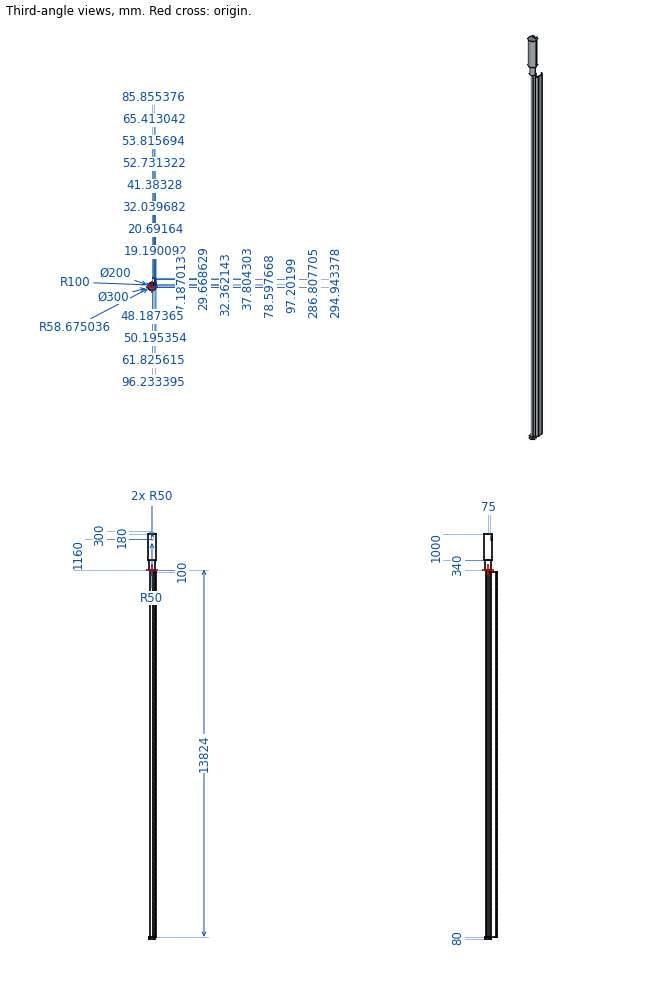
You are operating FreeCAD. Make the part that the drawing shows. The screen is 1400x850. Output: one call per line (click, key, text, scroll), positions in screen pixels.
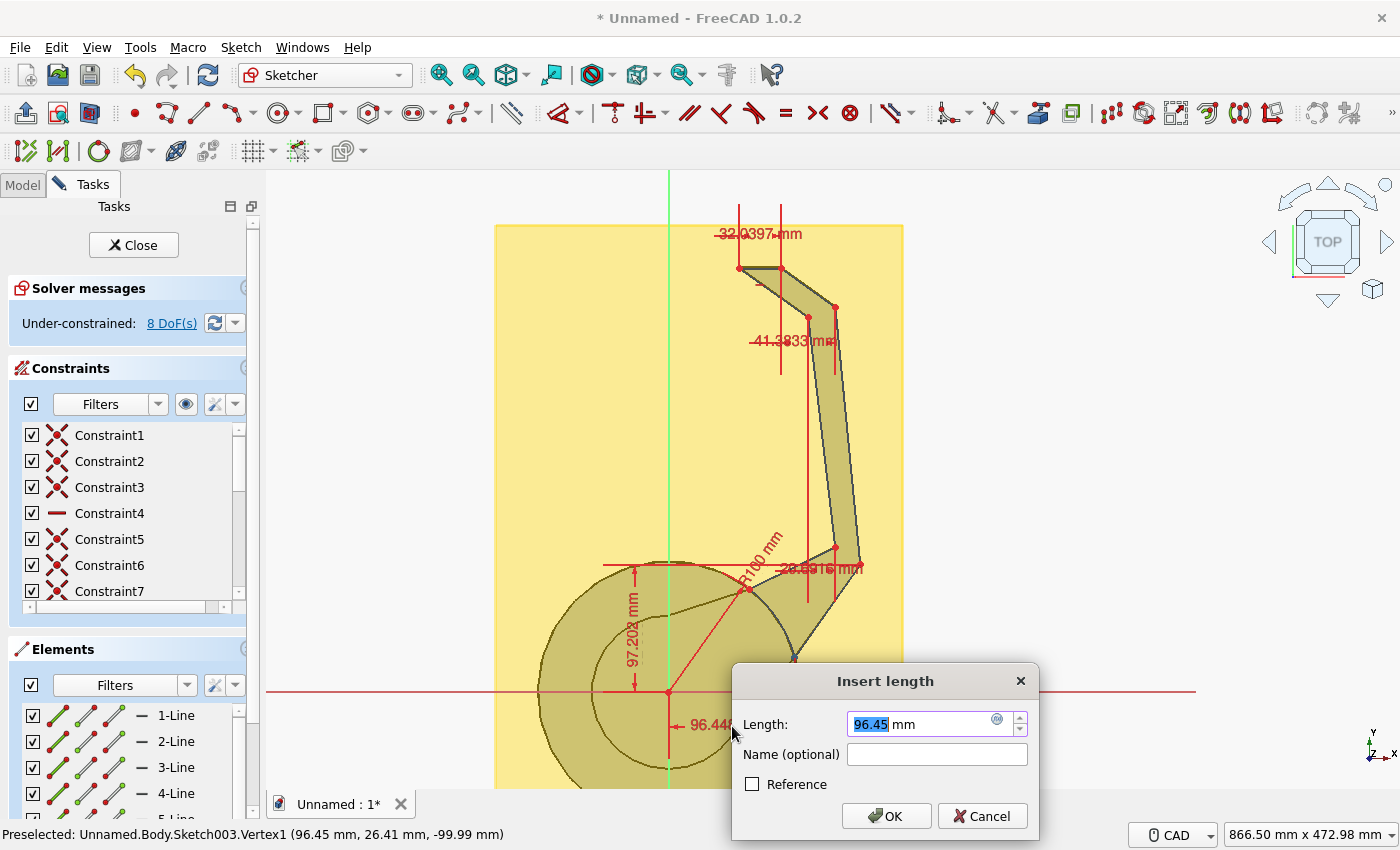
text(96.233395)
key(Return)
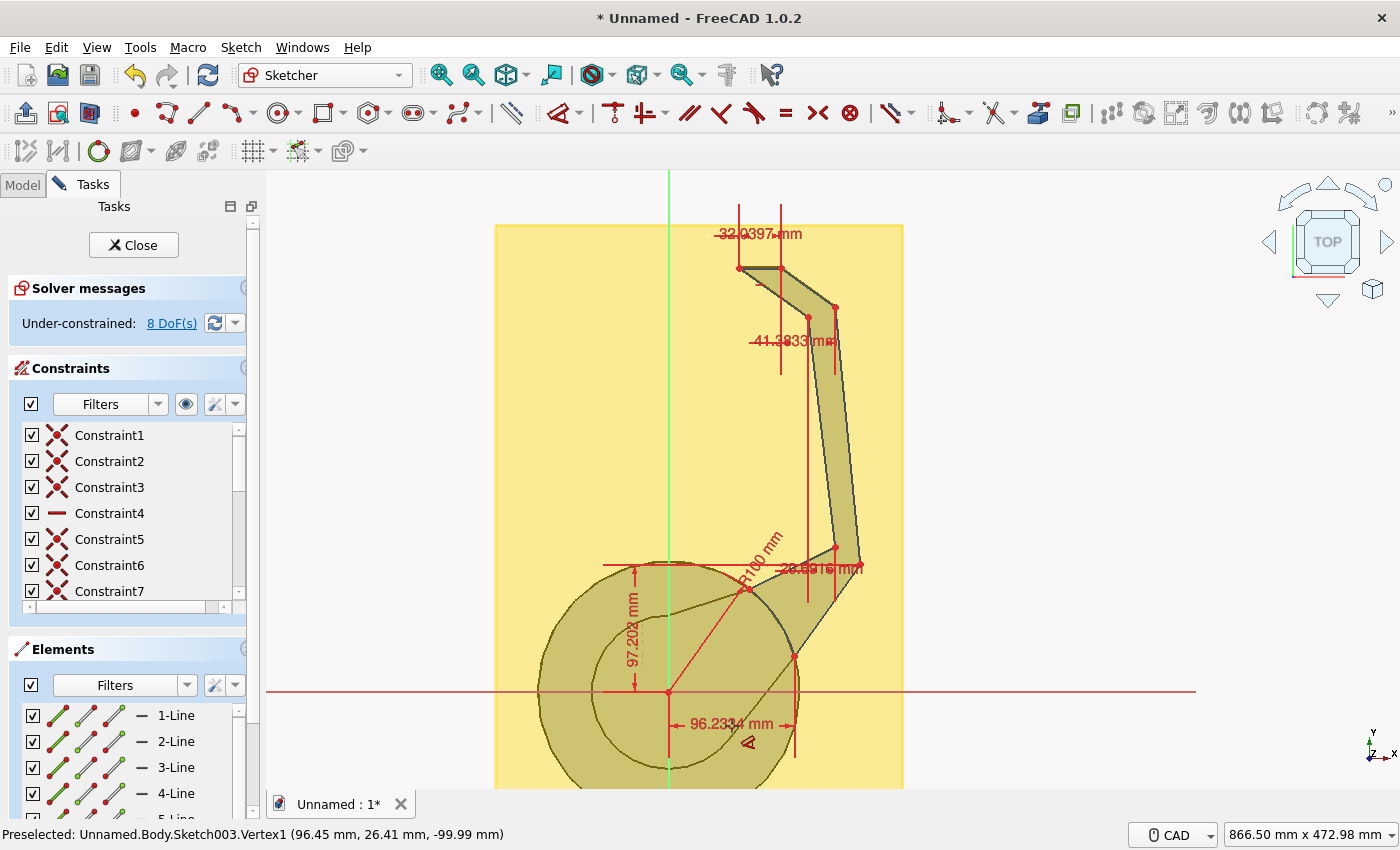
click(781, 269)
click(686, 235)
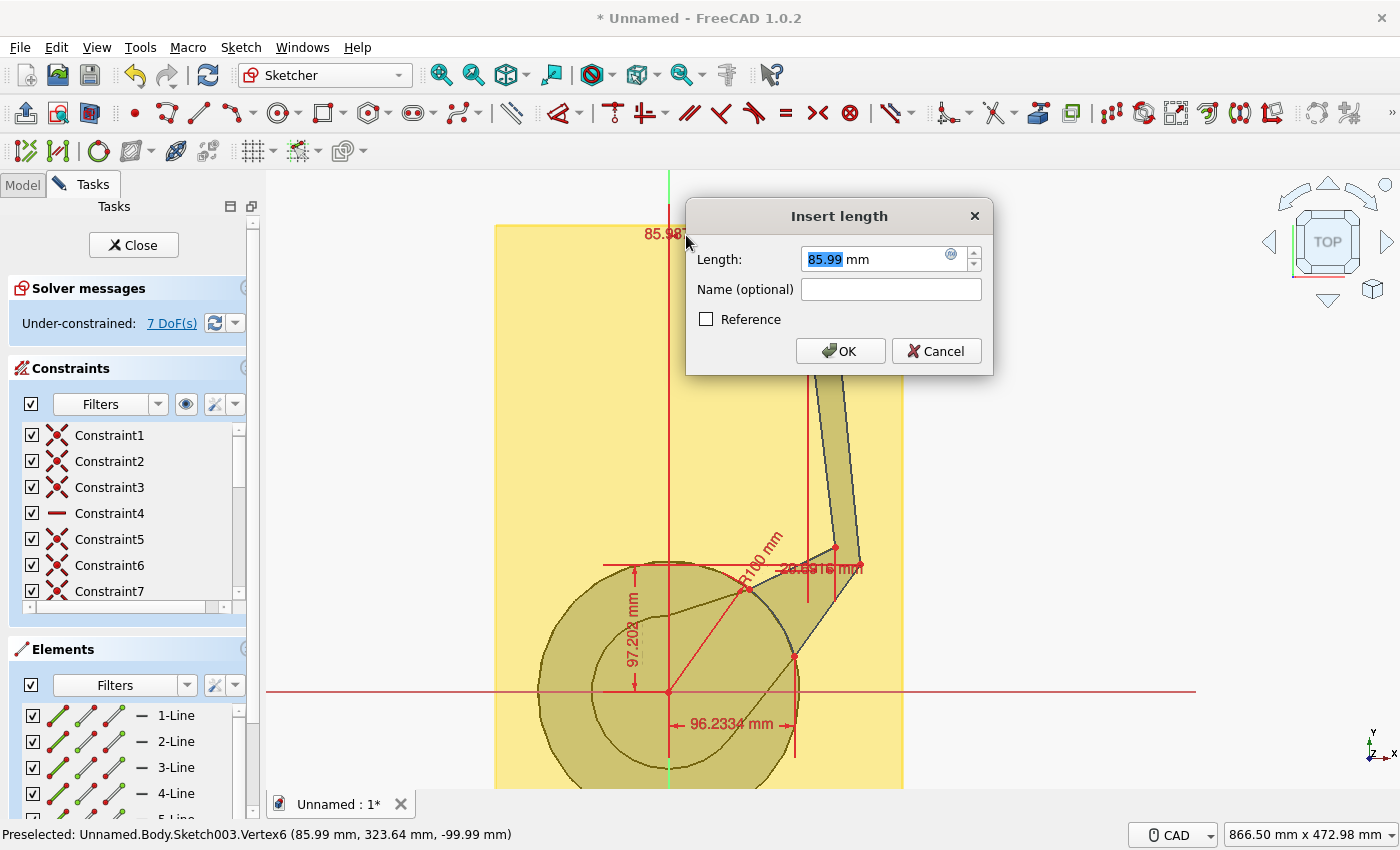
text(85.855376)
key(Return)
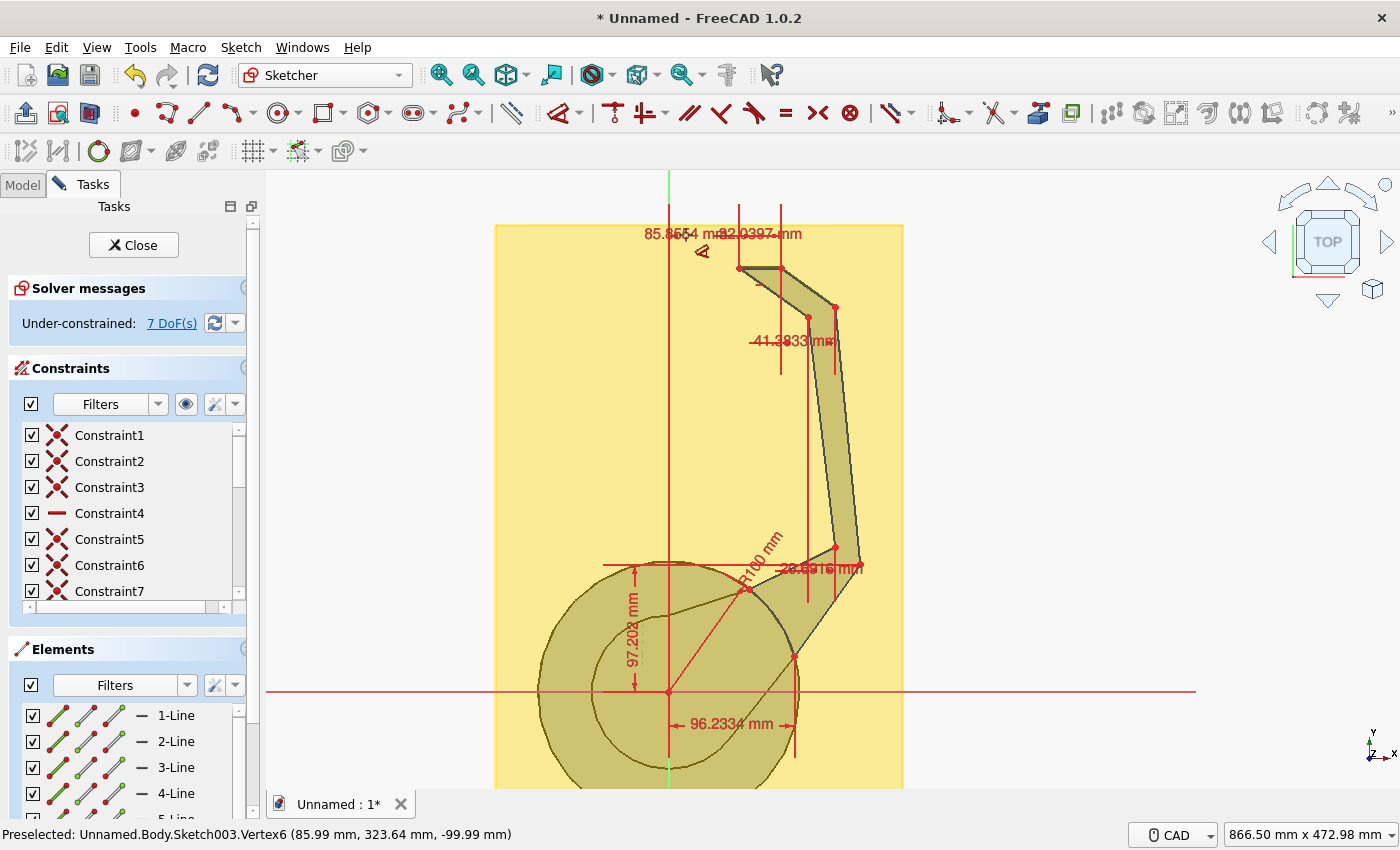
click(749, 589)
click(690, 555)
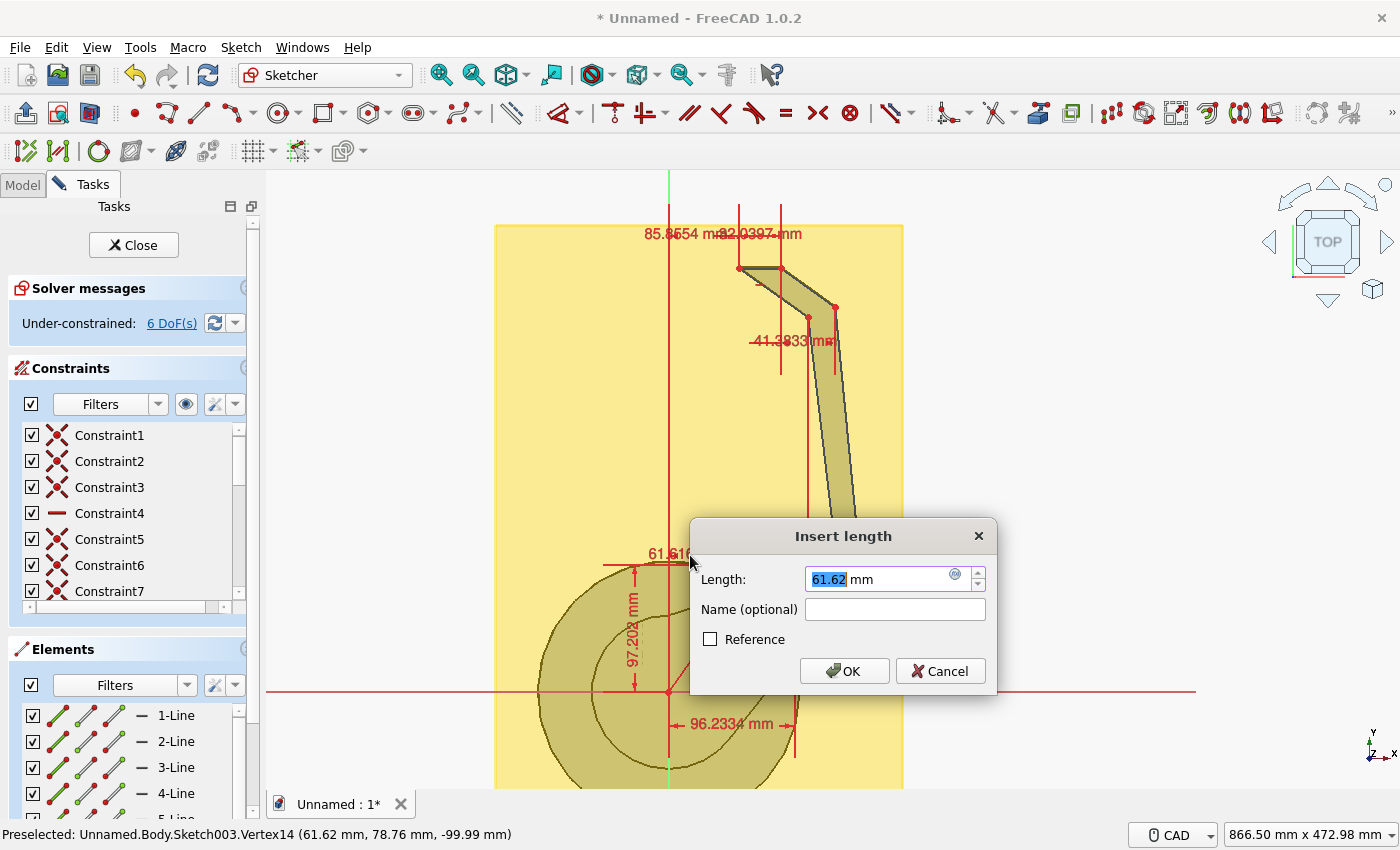
text(61.825615)
key(Return)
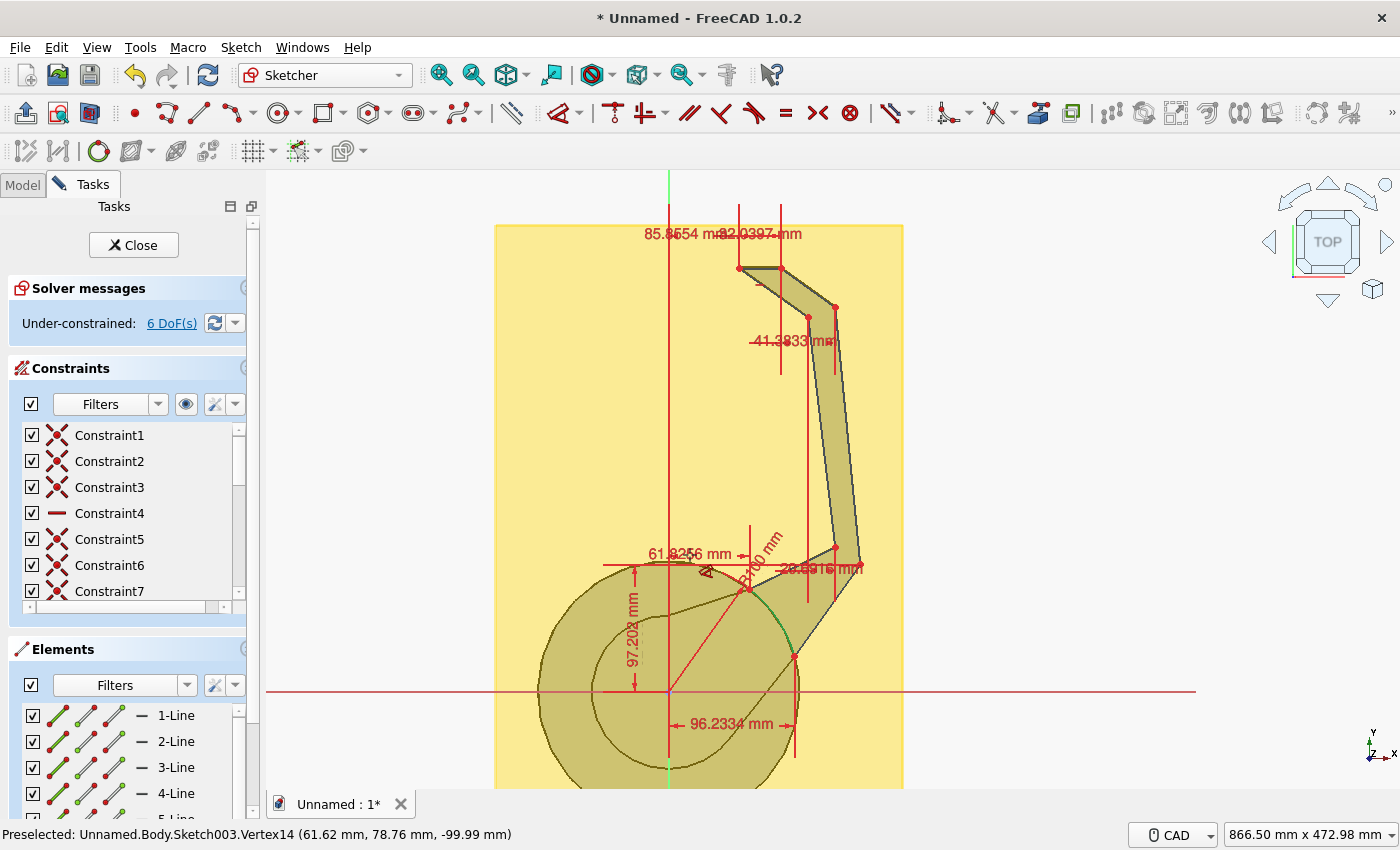
click(814, 629)
click(812, 531)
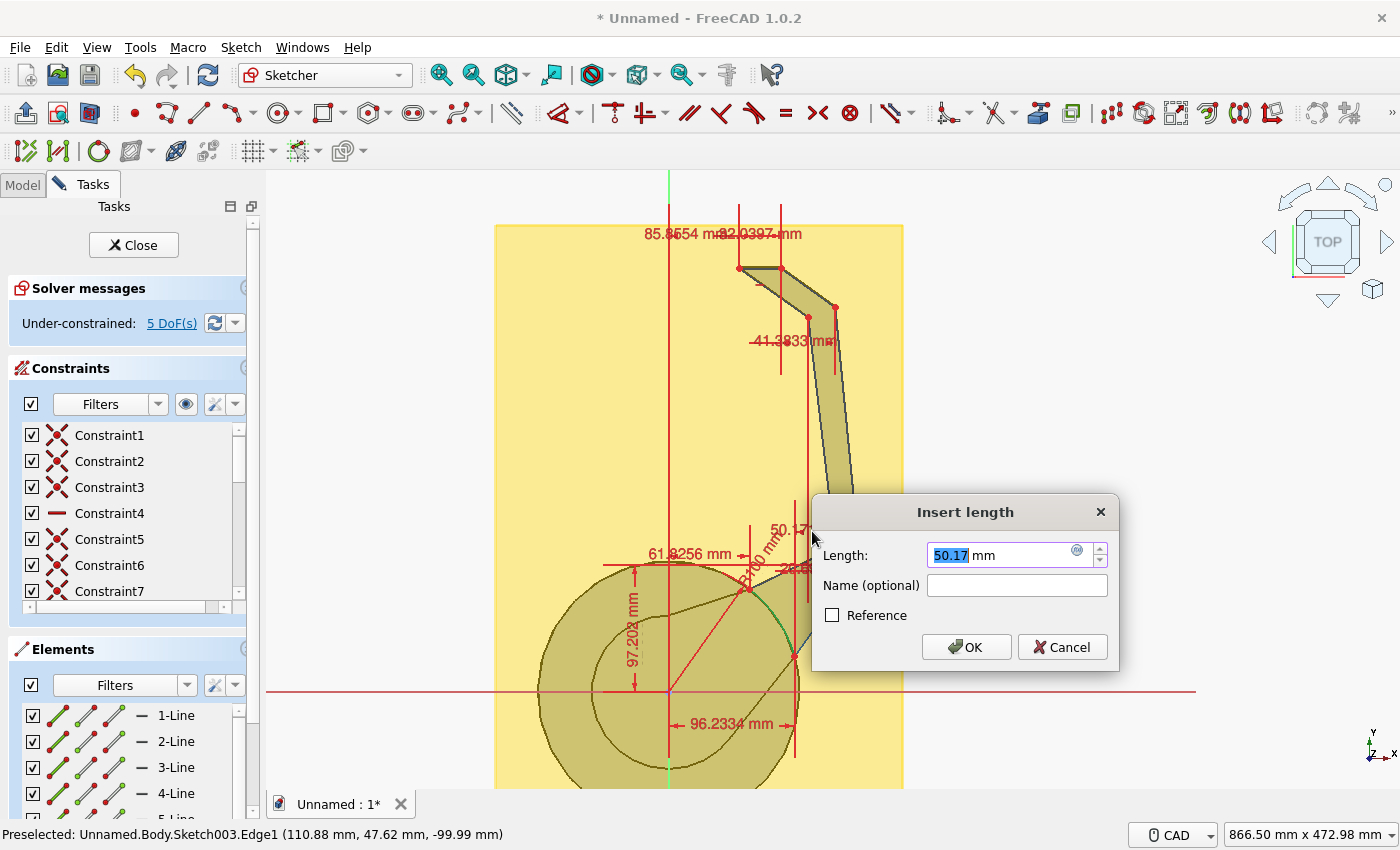
text(50.195354)
key(Return)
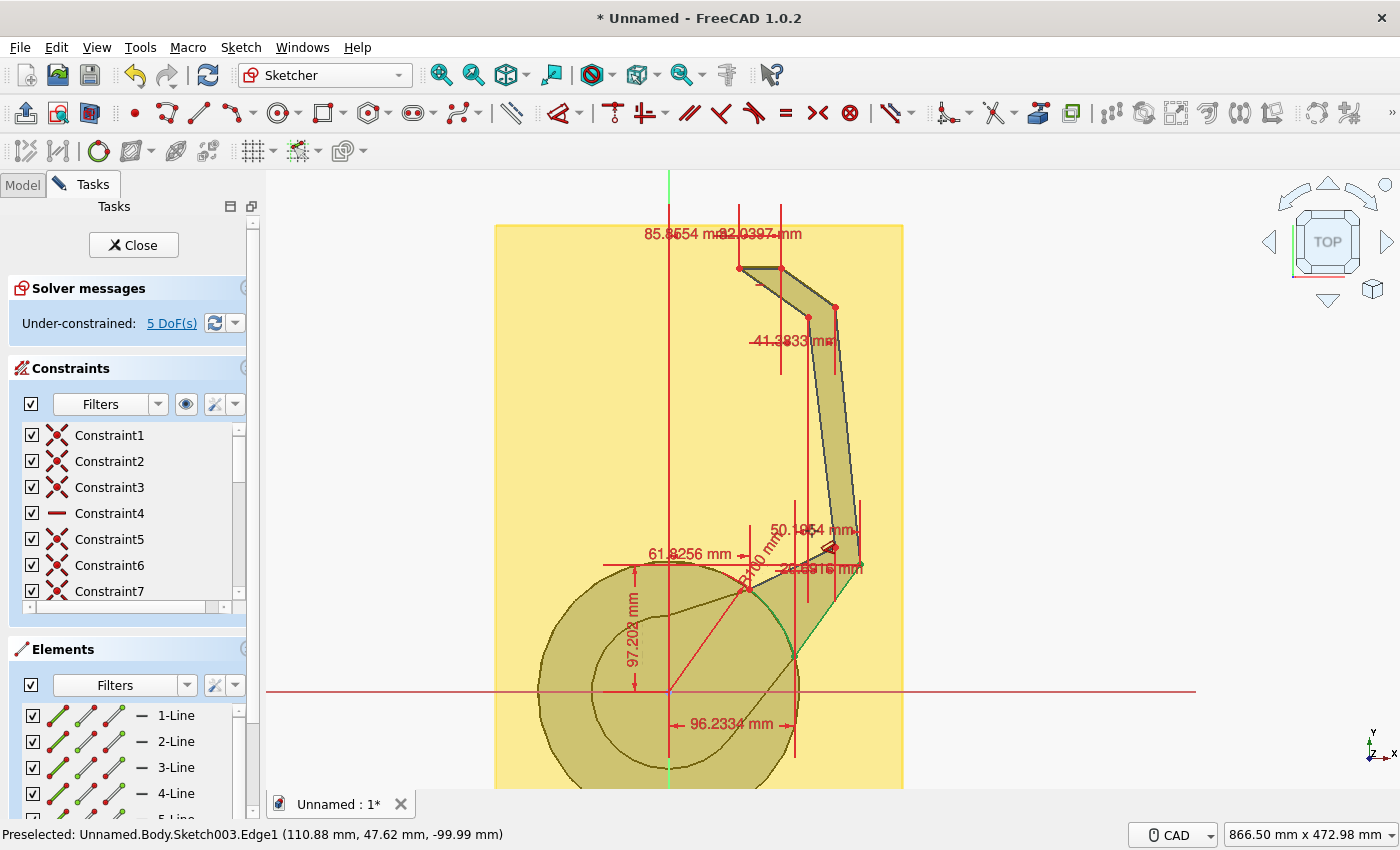
click(819, 296)
click(869, 288)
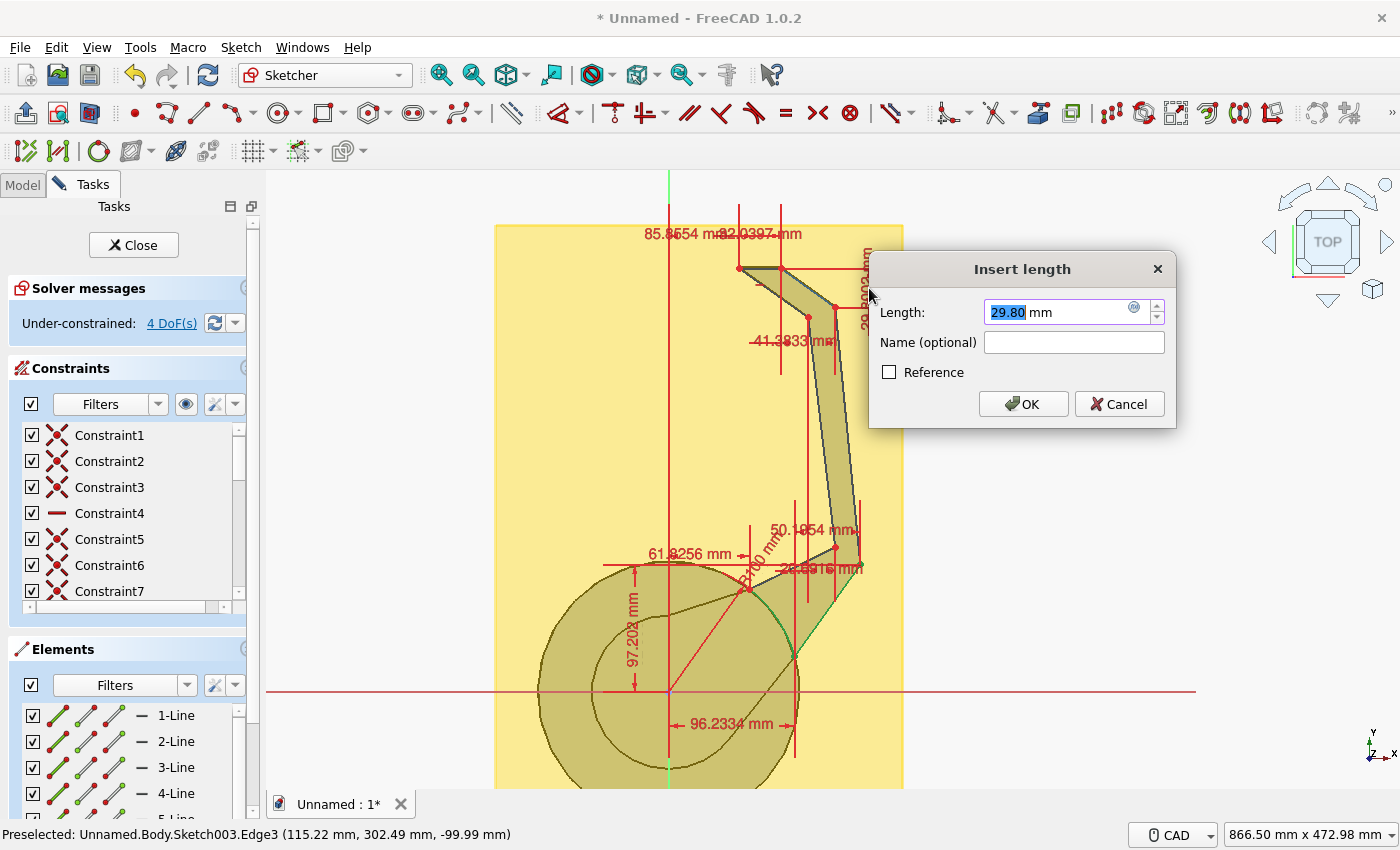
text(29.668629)
key(Return)